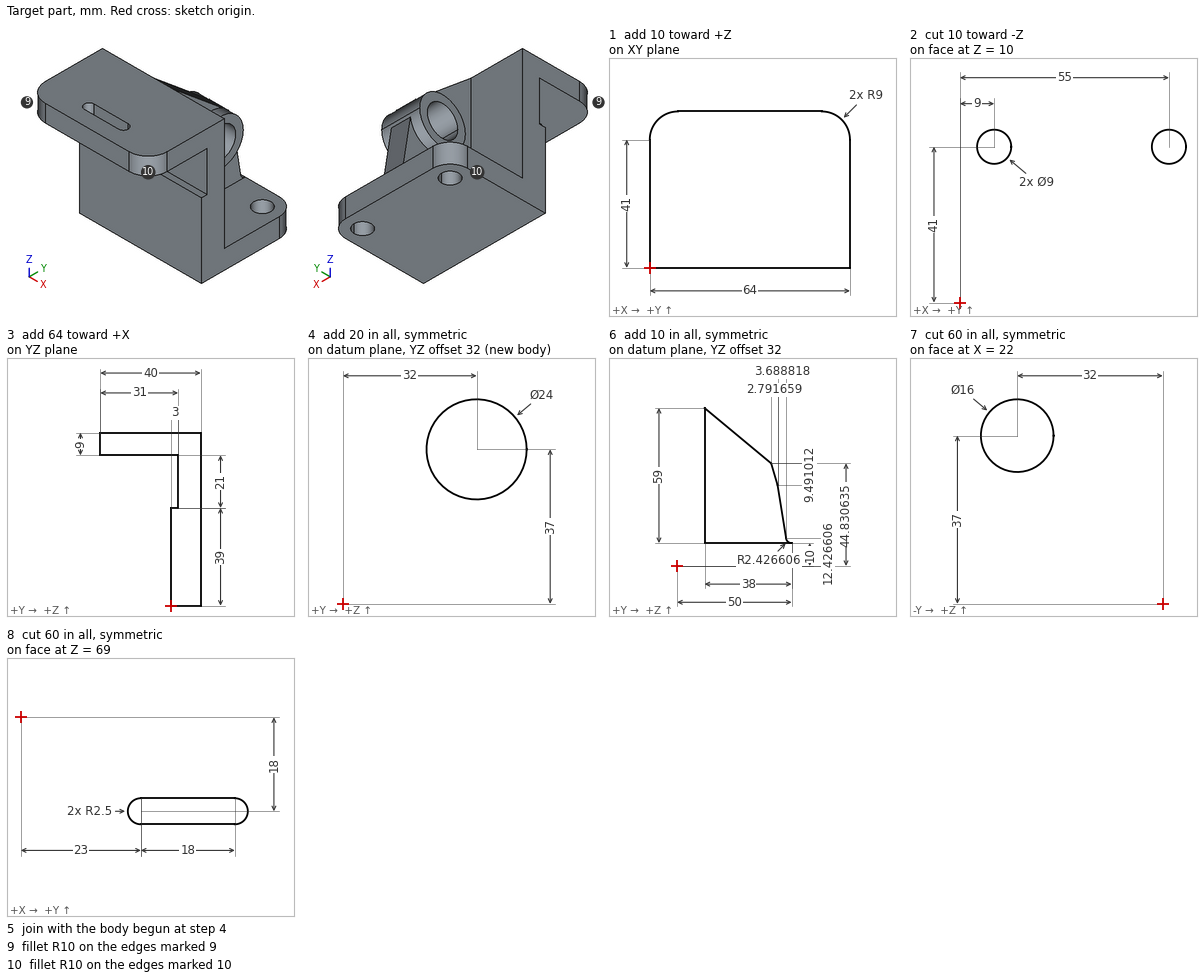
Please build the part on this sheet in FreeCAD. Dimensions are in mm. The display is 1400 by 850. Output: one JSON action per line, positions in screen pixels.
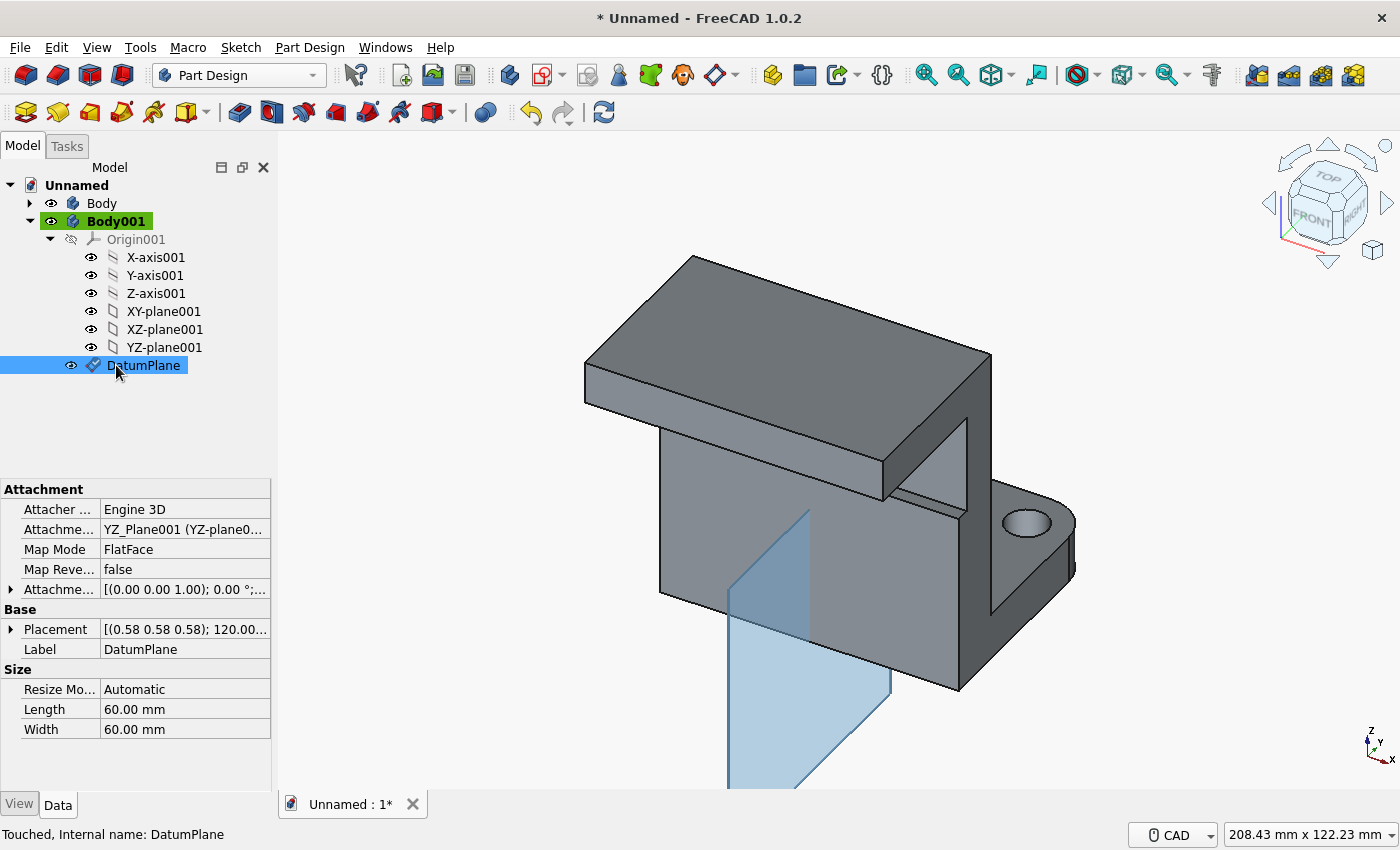
{"action": "left_click", "coordinate": [542, 76]}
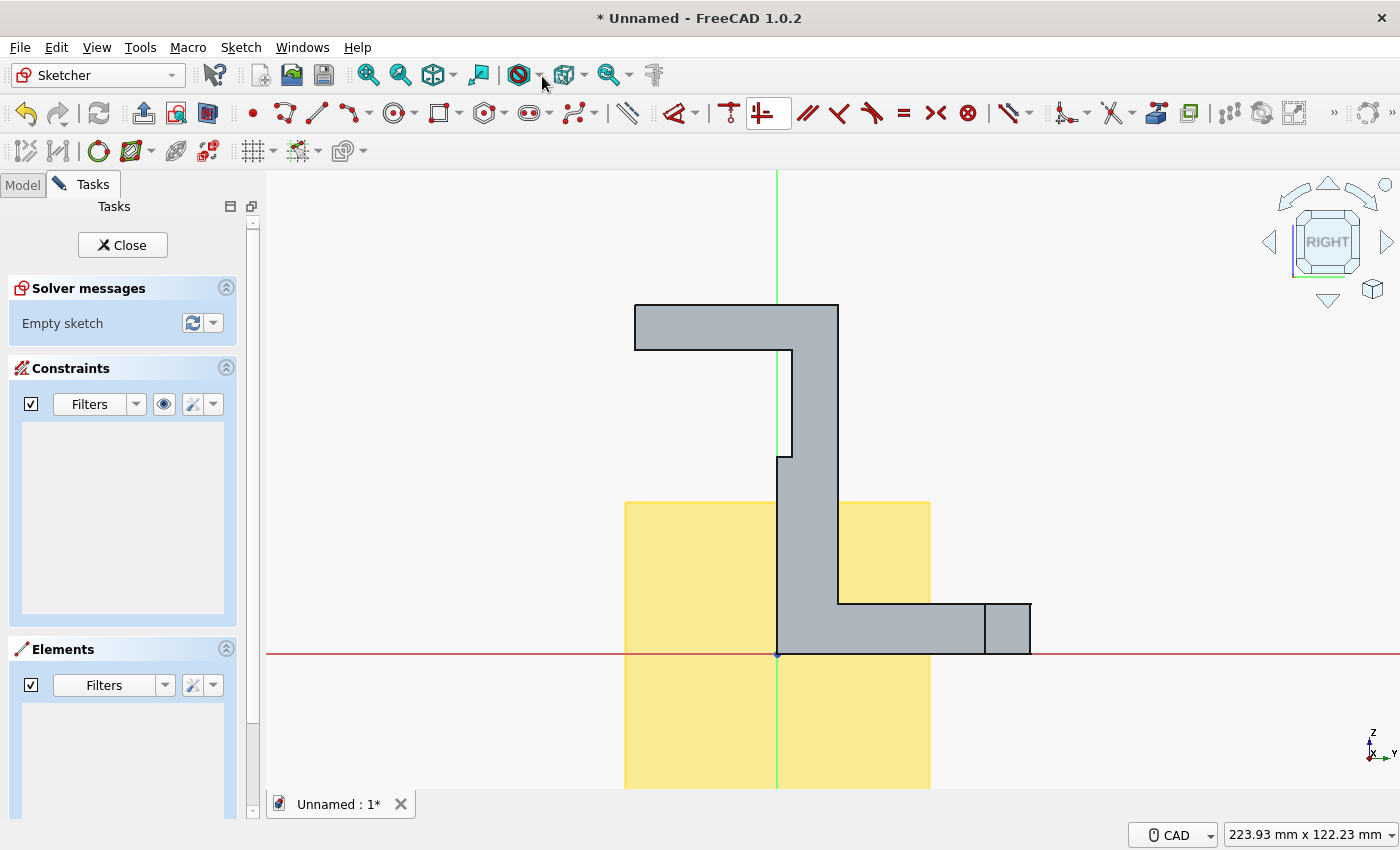
{"action": "scroll", "coordinate": [1141, 633], "scroll_direction": "up", "scroll_amount": 2}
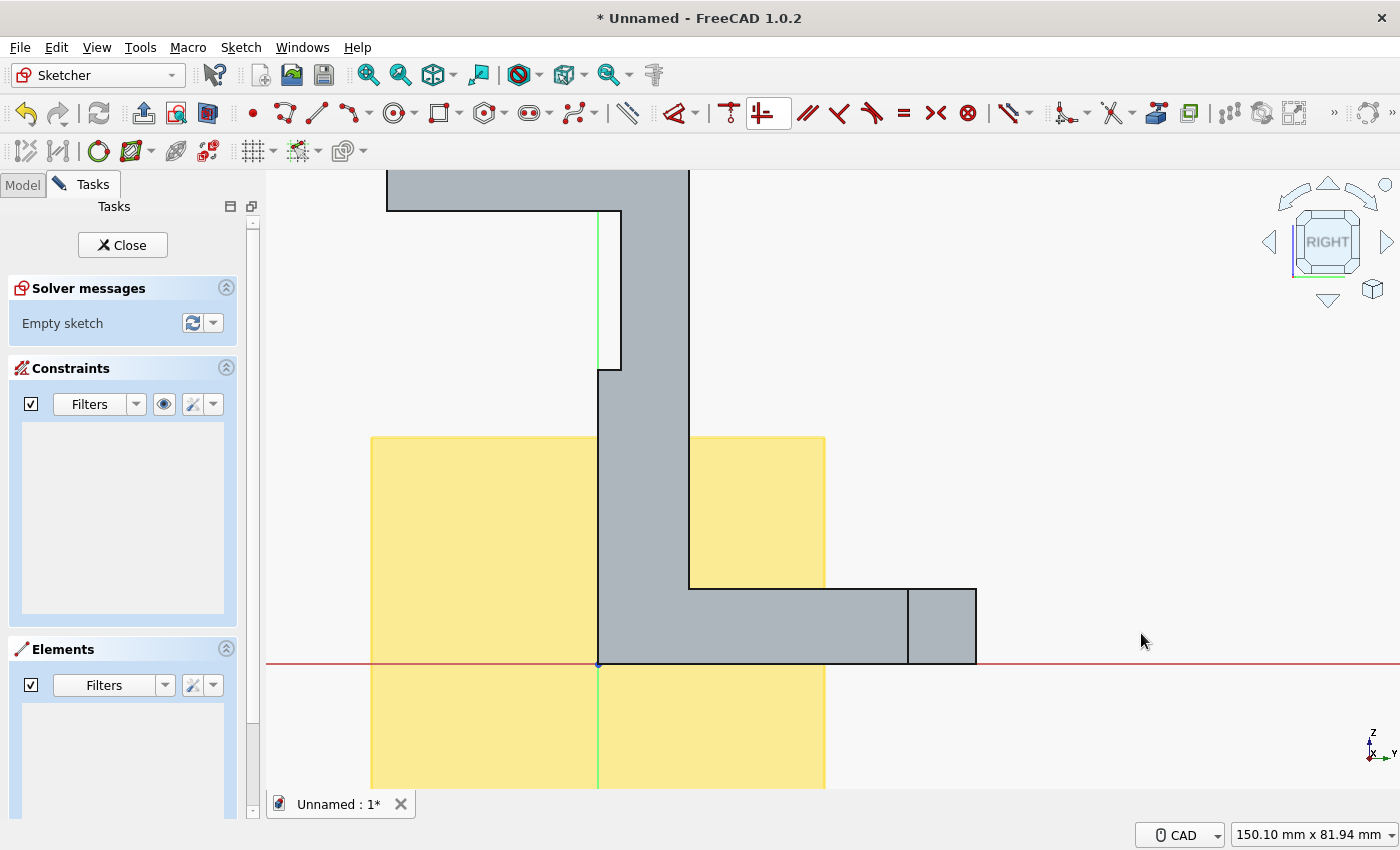
{"action": "left_click", "coordinate": [394, 114]}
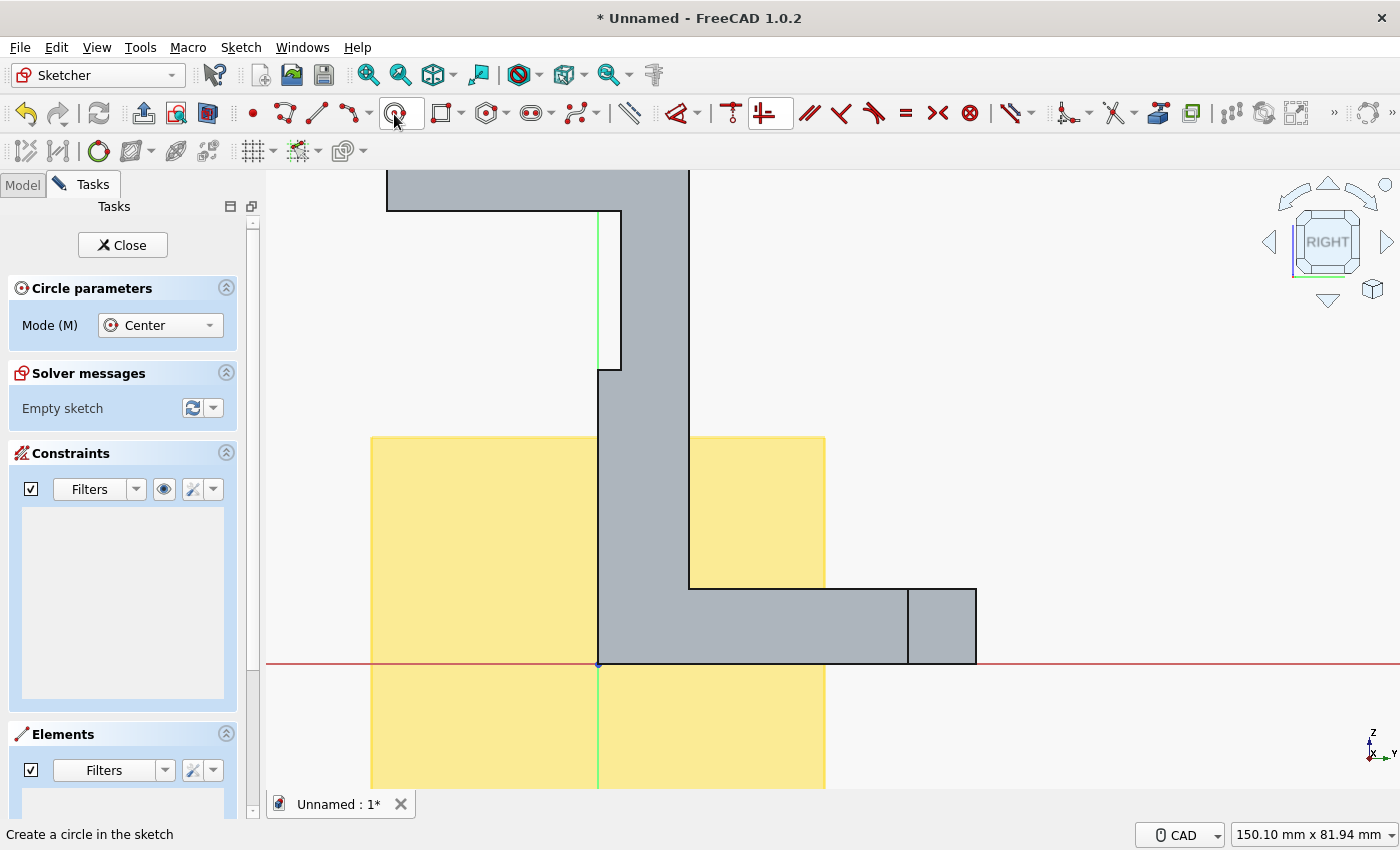
{"action": "left_click", "coordinate": [840, 385]}
{"action": "mouse_move", "coordinate": [904, 321]}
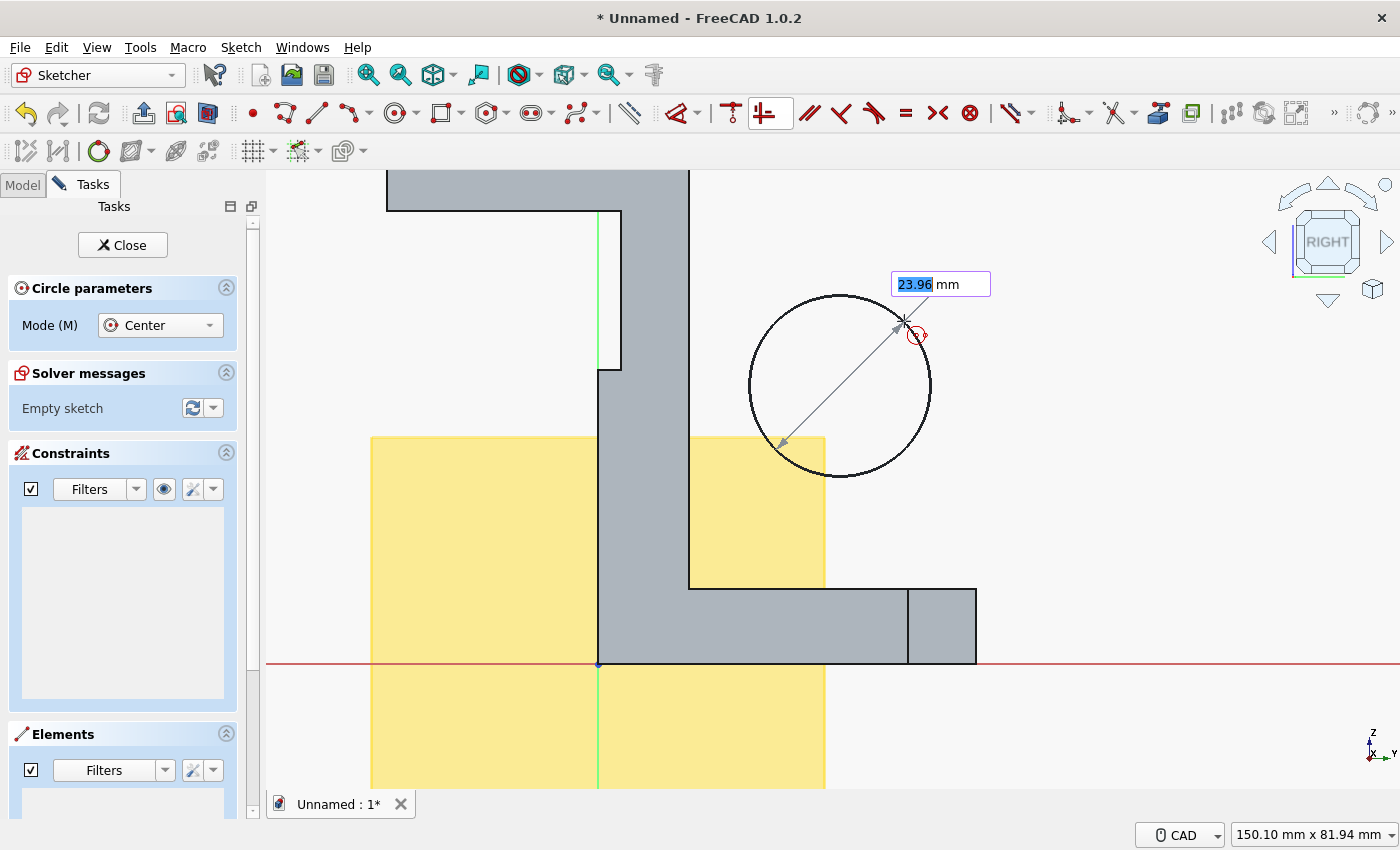
{"action": "type", "text": "24"}
{"action": "key", "text": "Return"}
{"action": "key", "text": "Escape"}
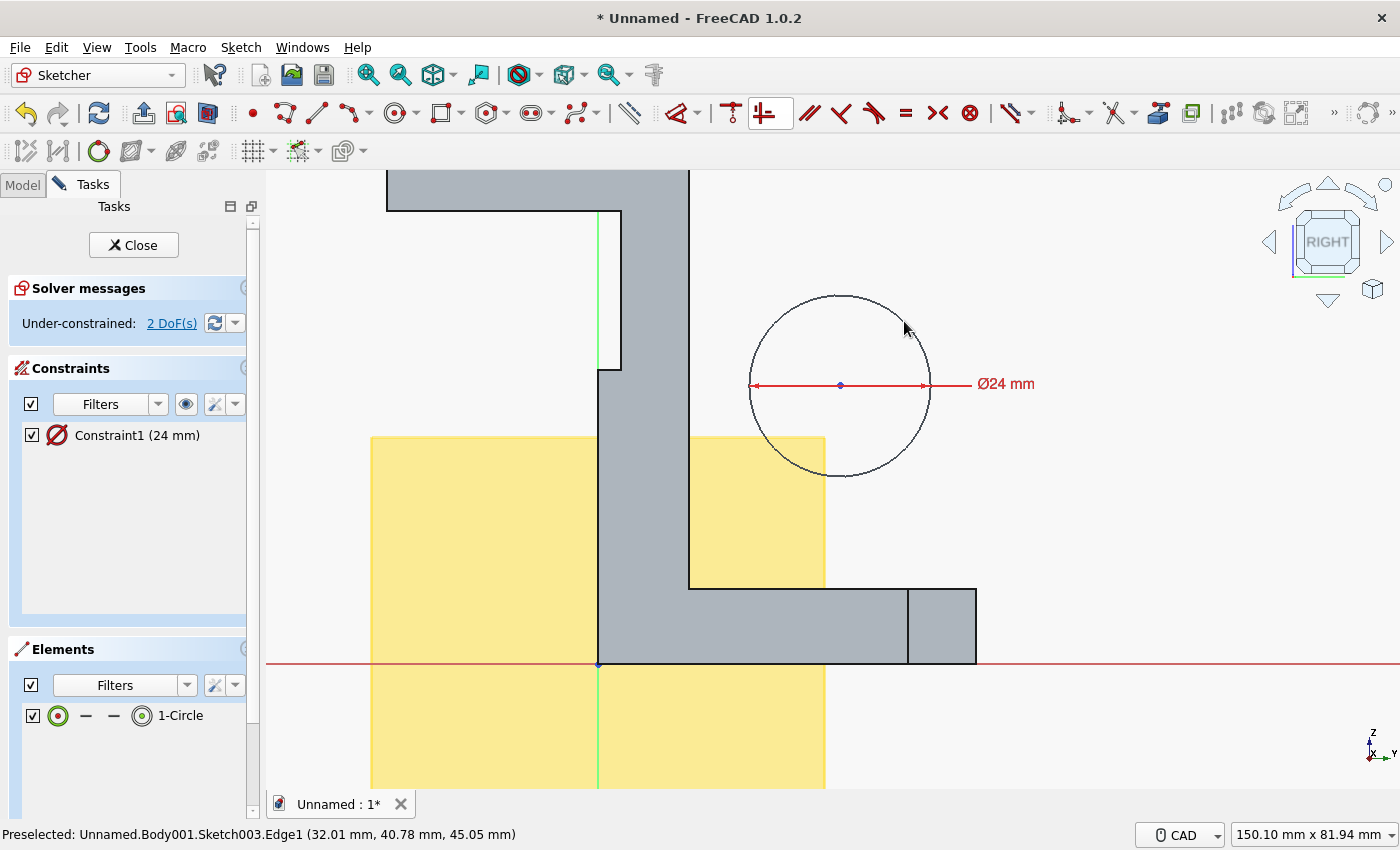
{"action": "left_click", "coordinate": [676, 114]}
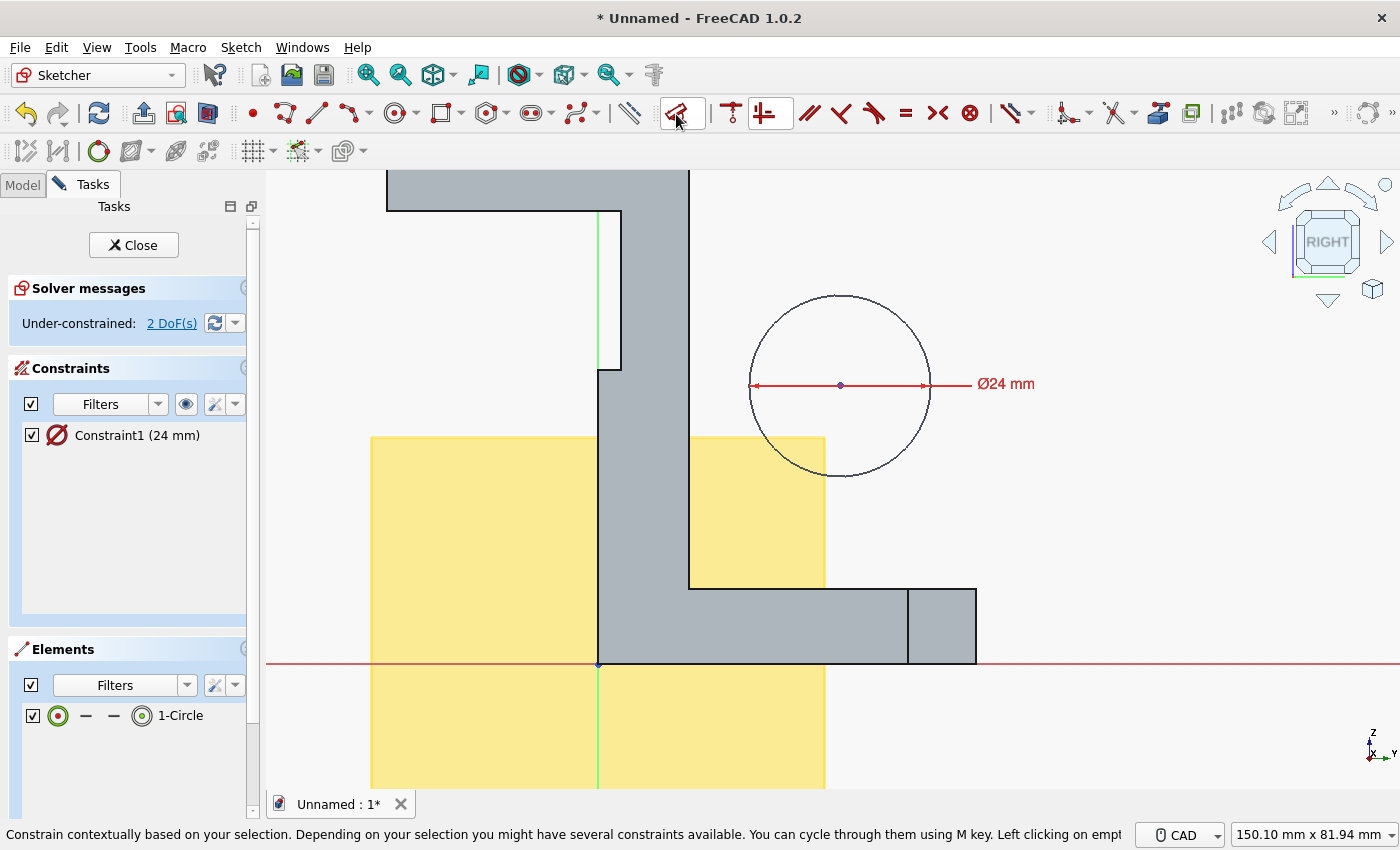
{"action": "left_click", "coordinate": [840, 386]}
{"action": "left_click", "coordinate": [719, 698]}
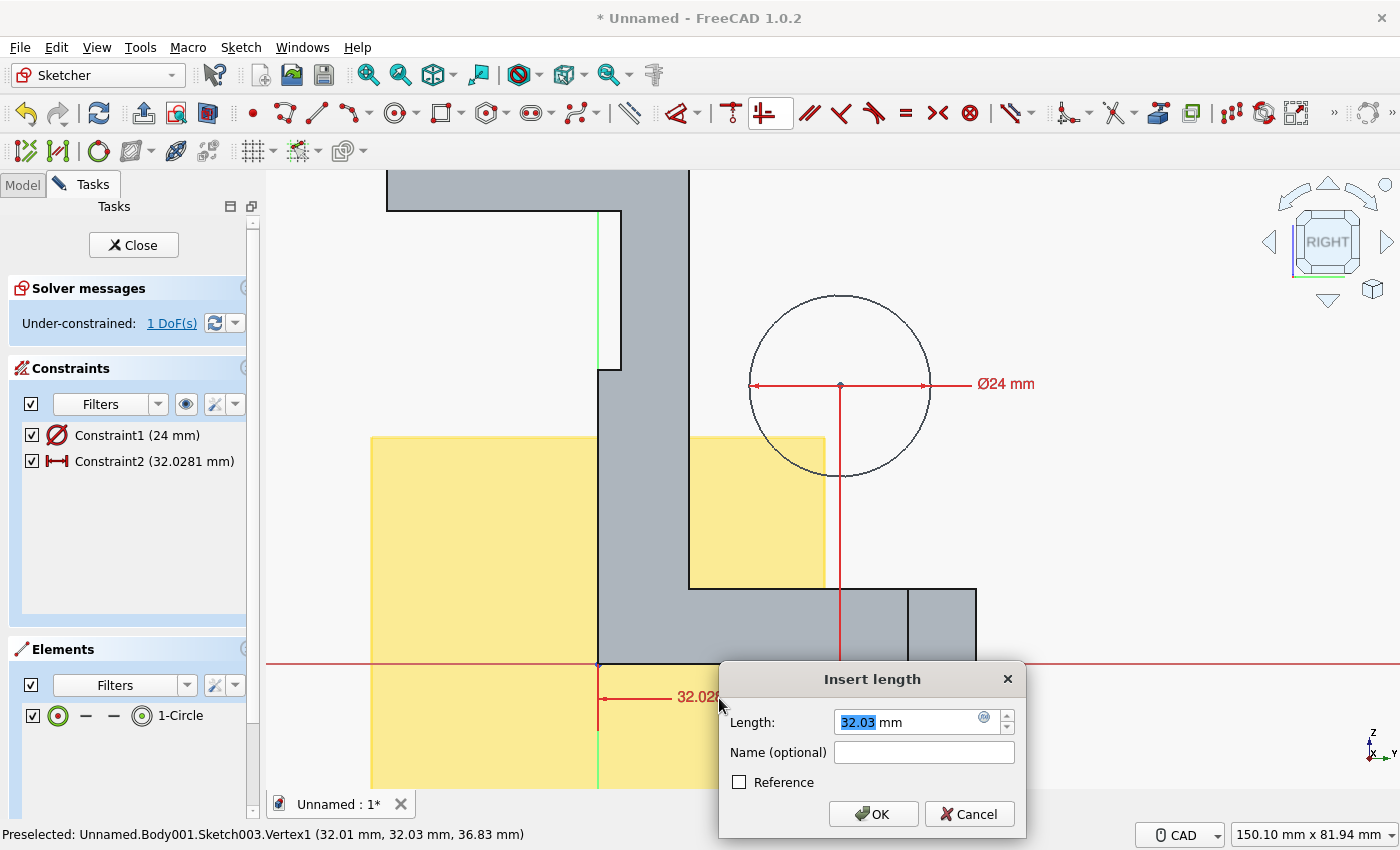
{"action": "type", "text": "32"}
{"action": "key", "text": "Return"}